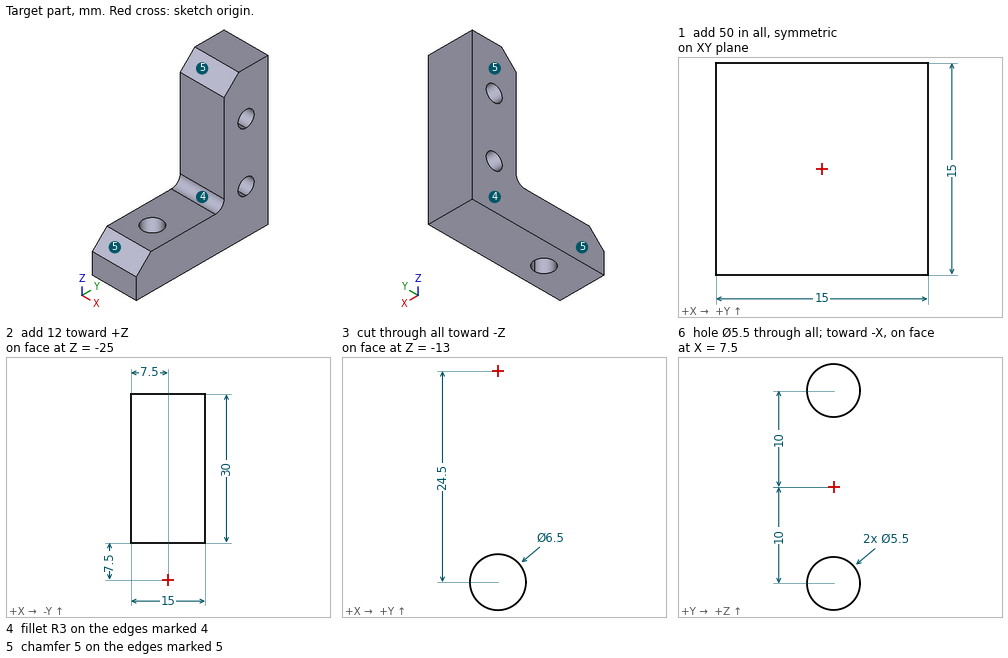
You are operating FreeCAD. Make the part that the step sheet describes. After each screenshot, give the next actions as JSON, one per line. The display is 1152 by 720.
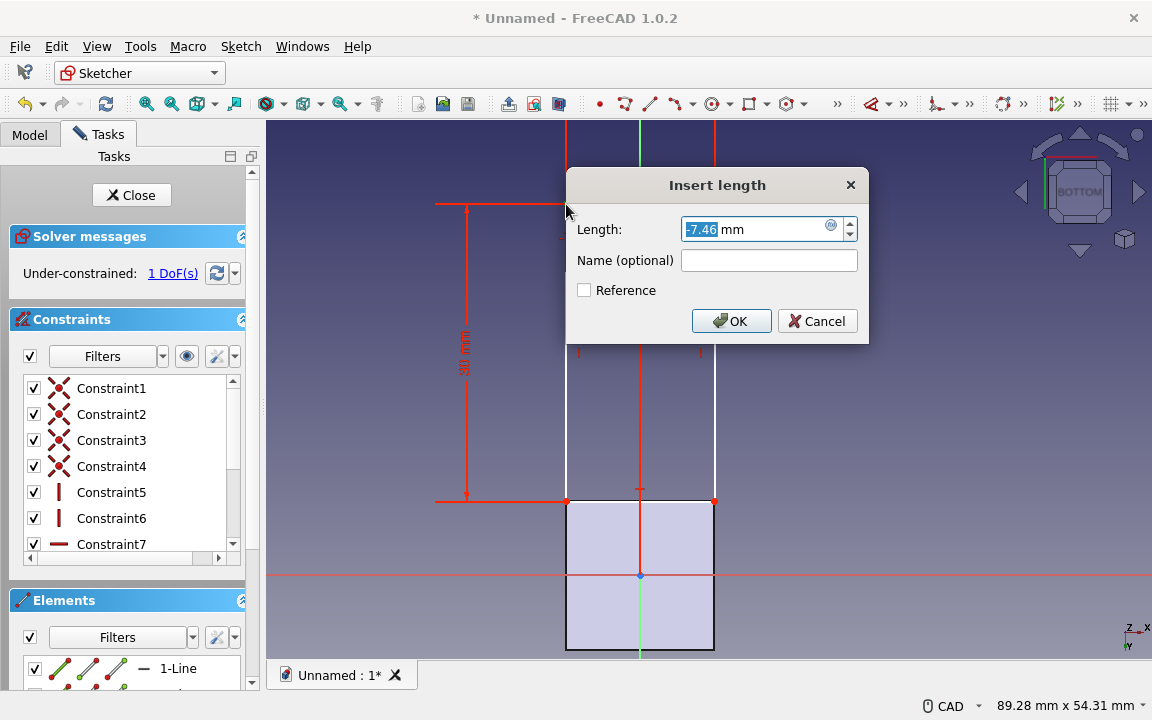
{"action": "type", "text": "-7.5"}
{"action": "key", "text": "Return"}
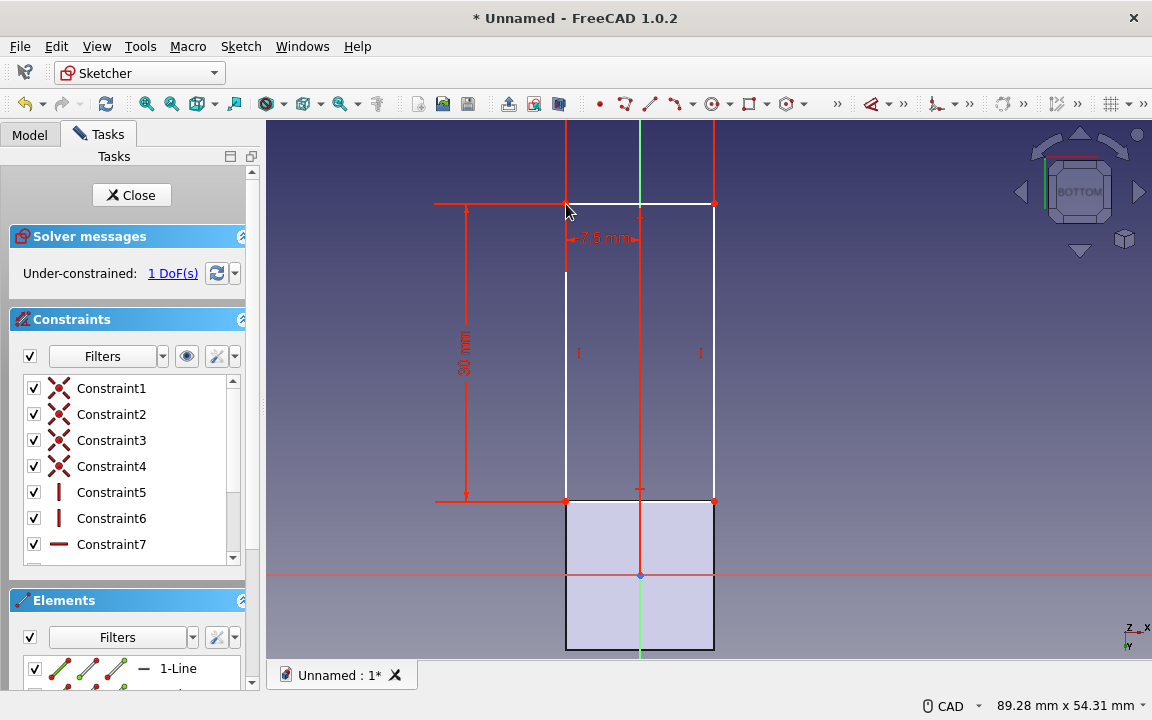
{"action": "left_click", "coordinate": [566, 502]}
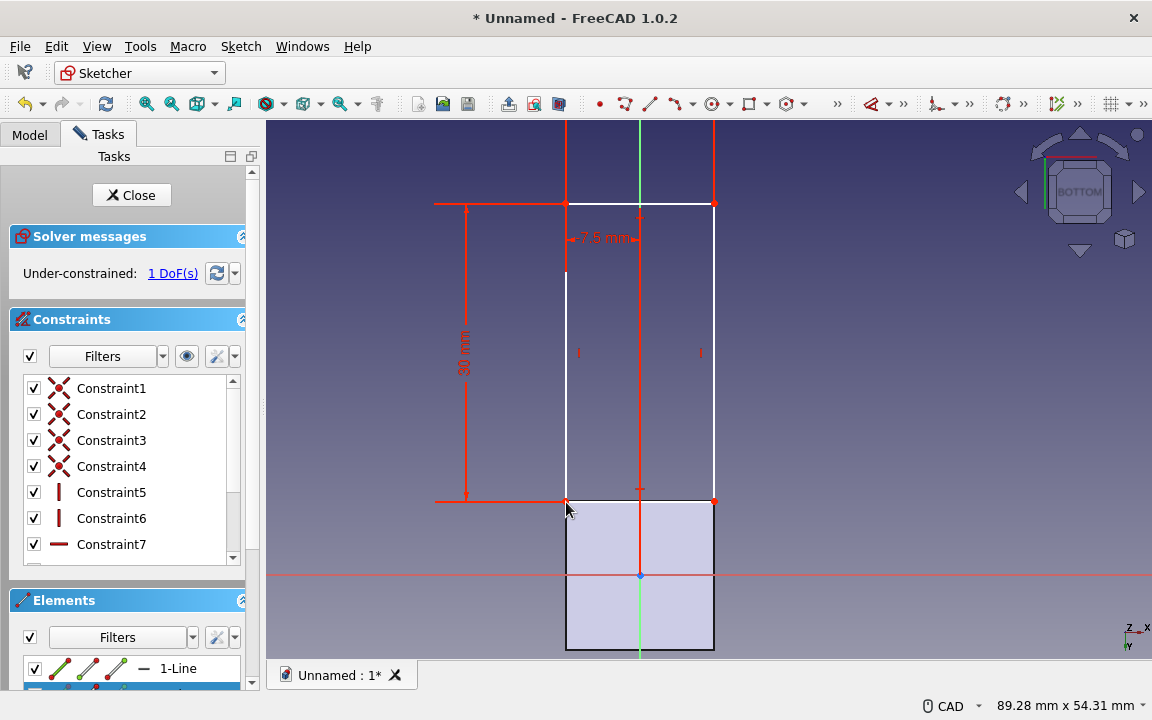
{"action": "key", "text": "i"}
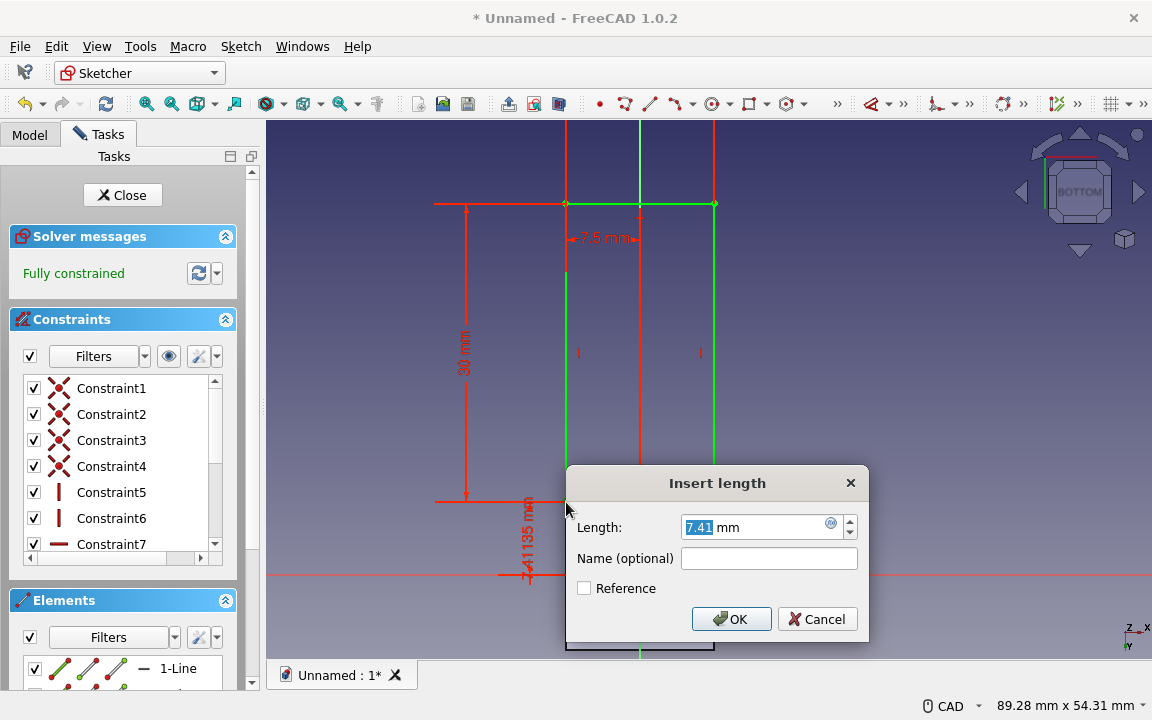
{"action": "type", "text": "7.5"}
{"action": "key", "text": "Return"}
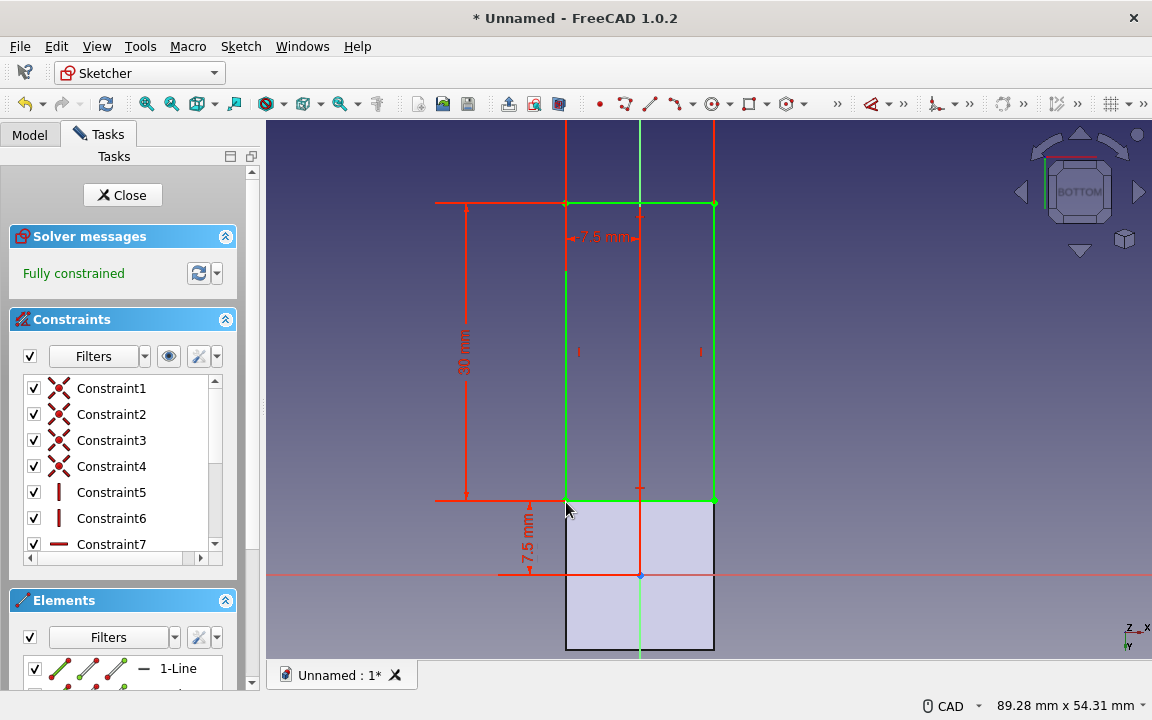
{"action": "left_click", "coordinate": [123, 195]}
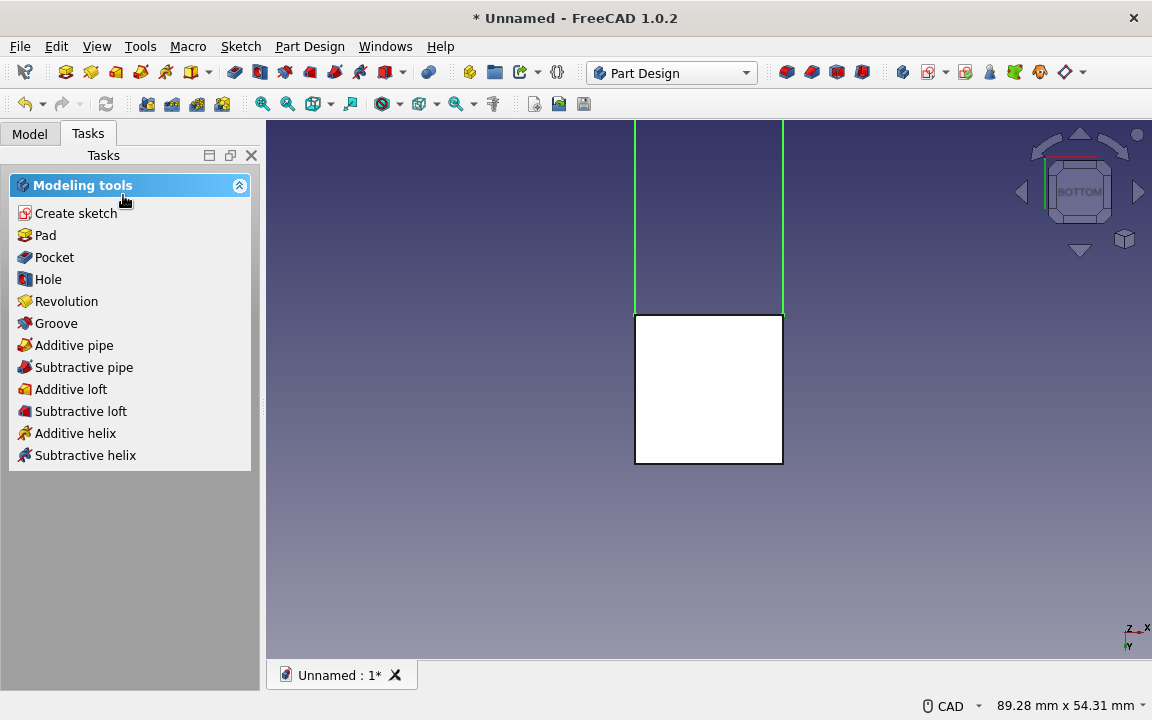
{"action": "left_click", "coordinate": [66, 72]}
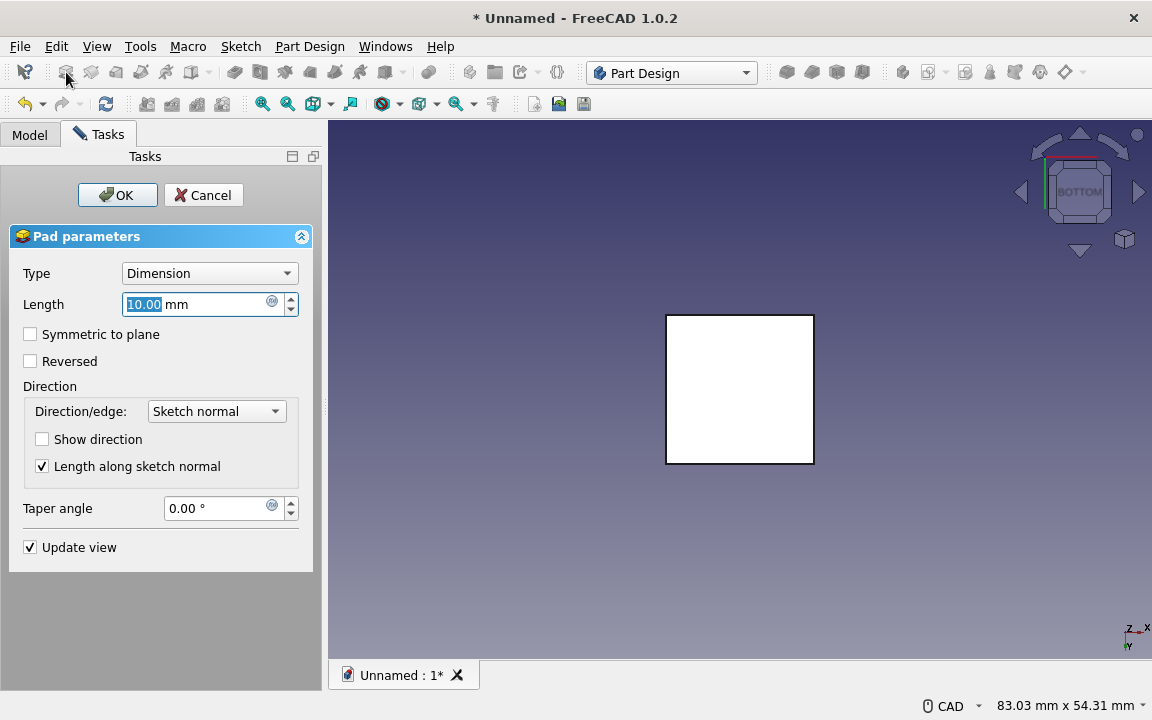
{"action": "type", "text": "12"}
{"action": "key", "text": "Tab"}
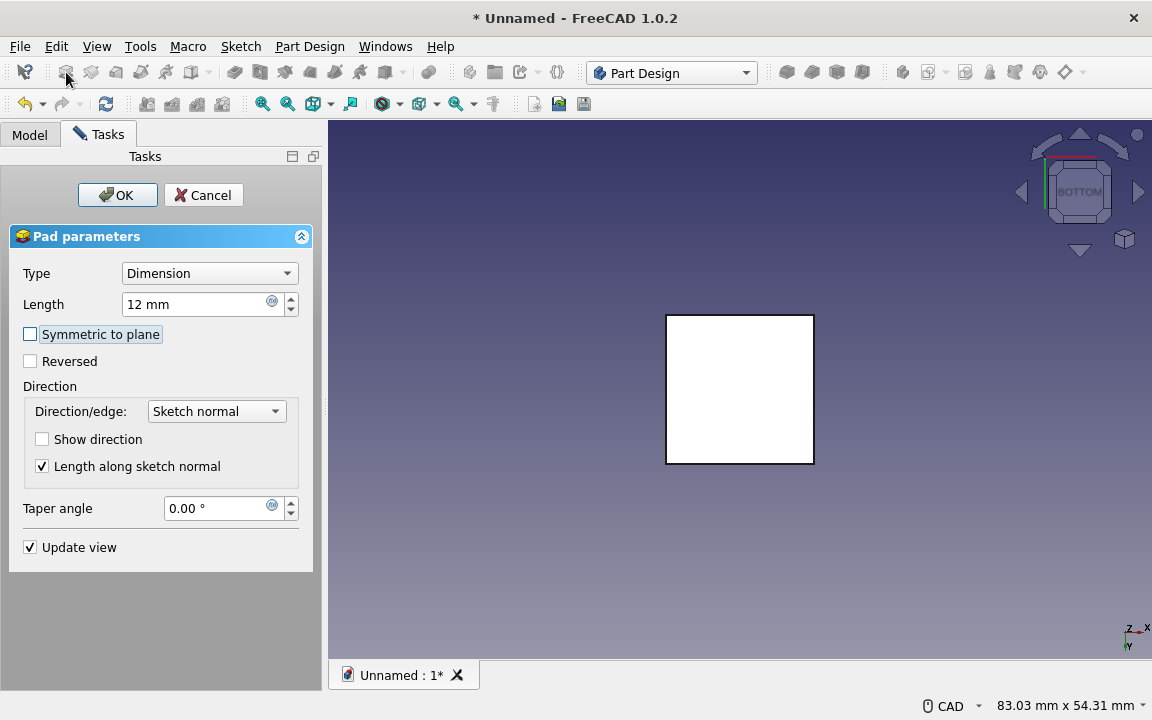
{"action": "left_click", "coordinate": [31, 361]}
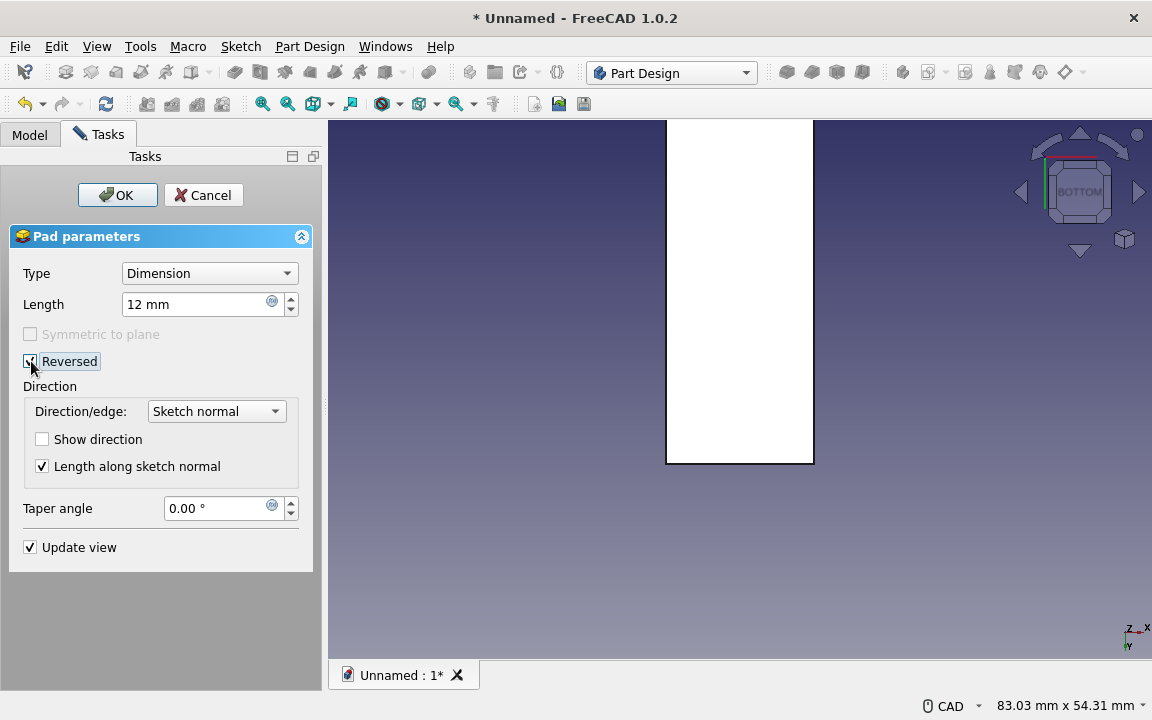
{"action": "left_click", "coordinate": [118, 195]}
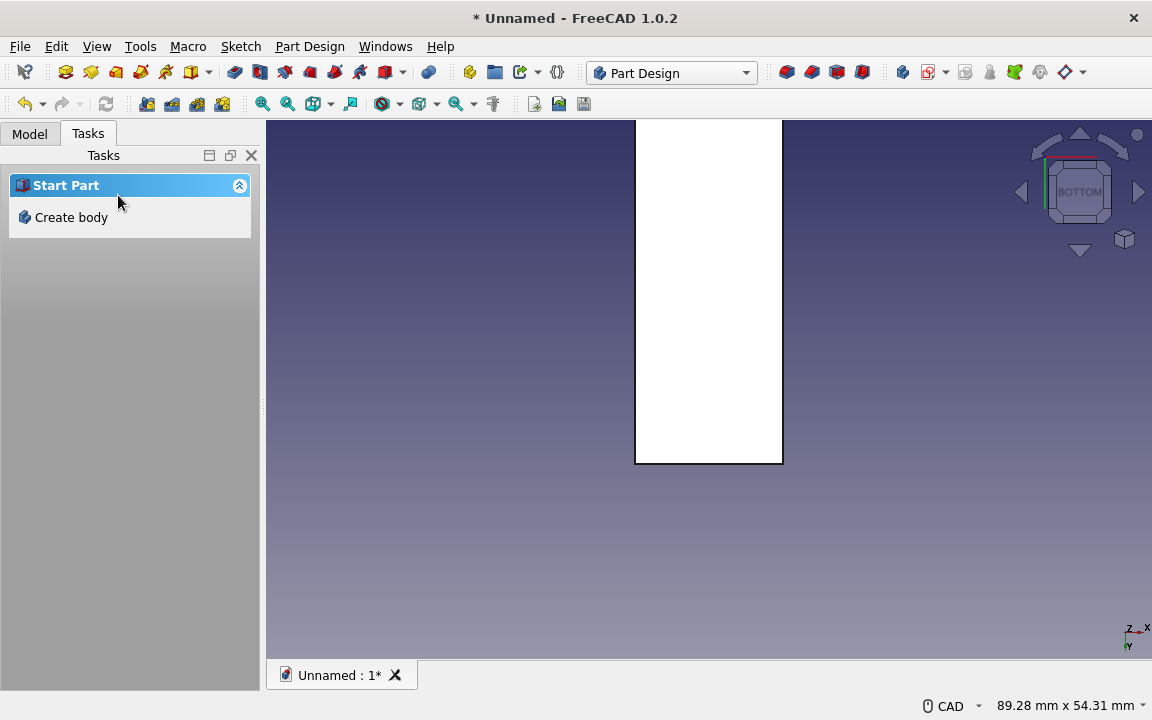
{"action": "key", "text": "v f"}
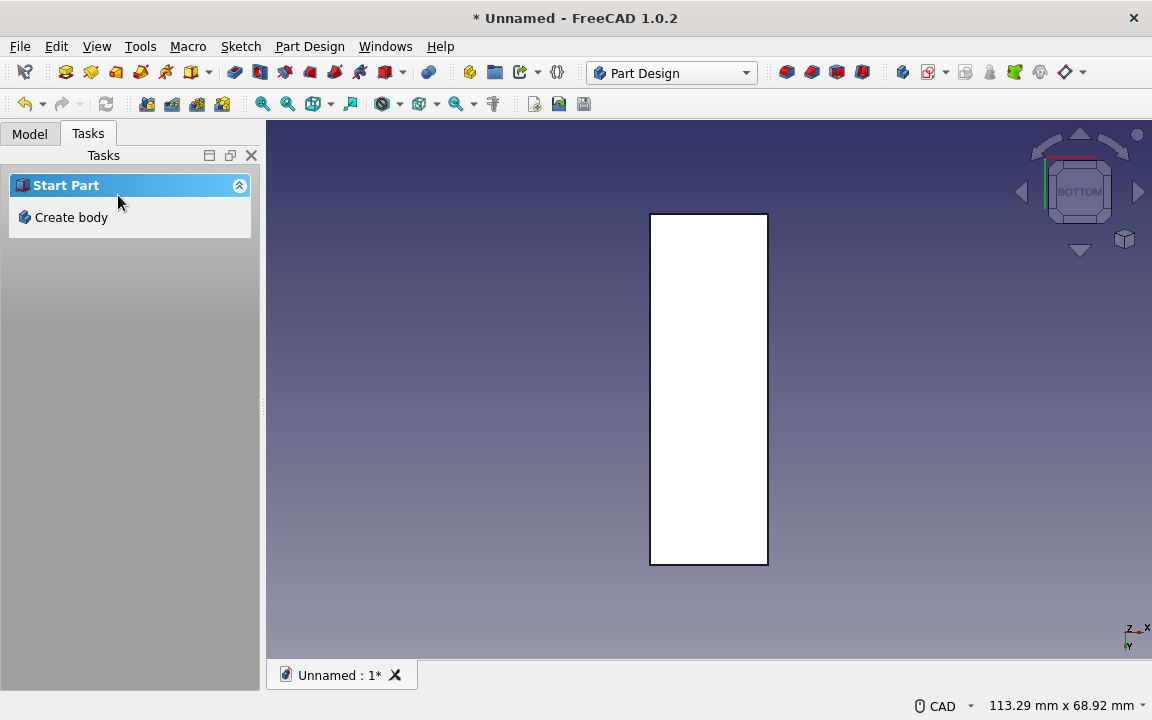
{"action": "key", "text": "0"}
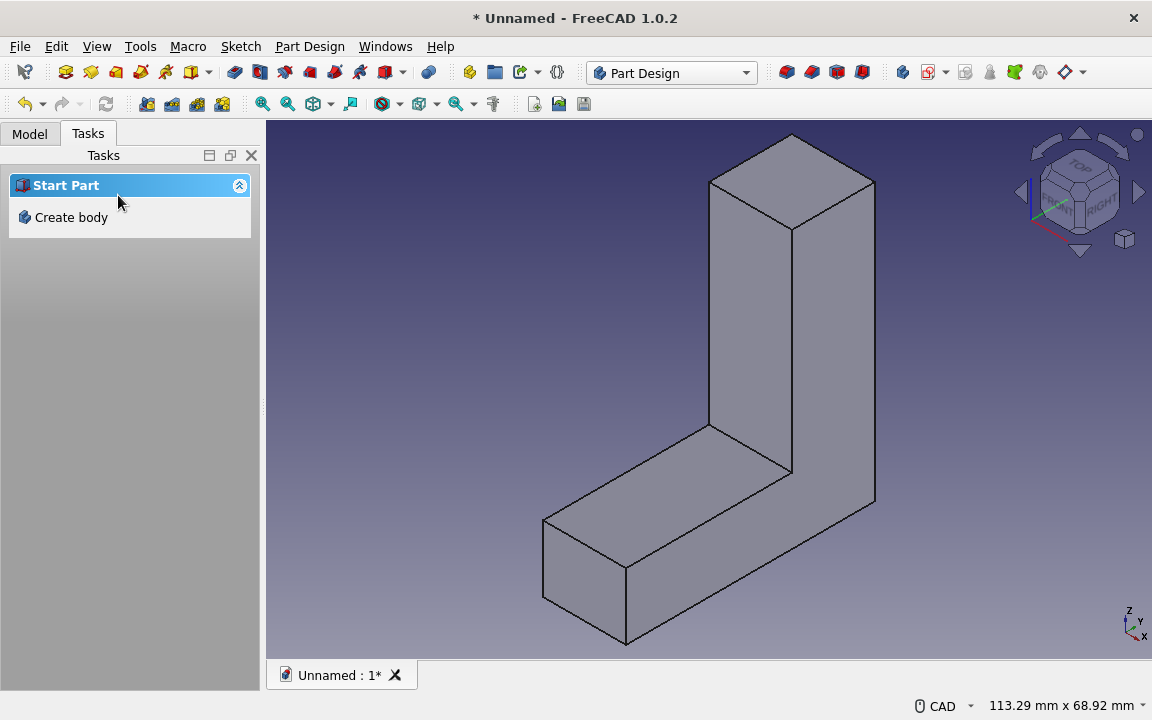
{"action": "left_click", "coordinate": [691, 482]}